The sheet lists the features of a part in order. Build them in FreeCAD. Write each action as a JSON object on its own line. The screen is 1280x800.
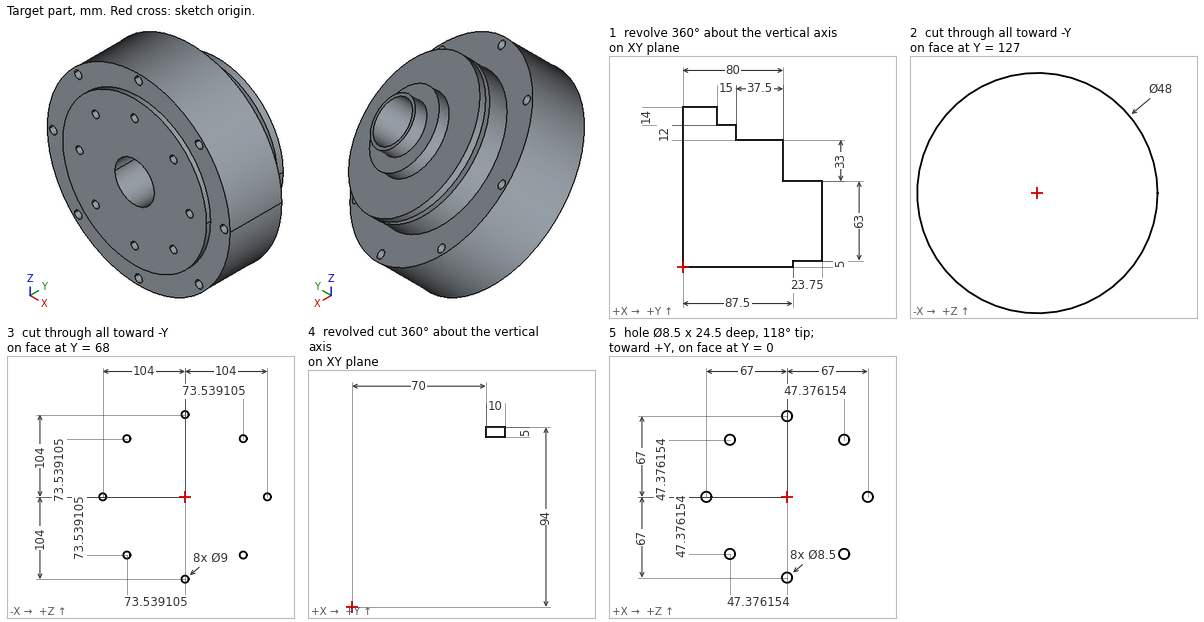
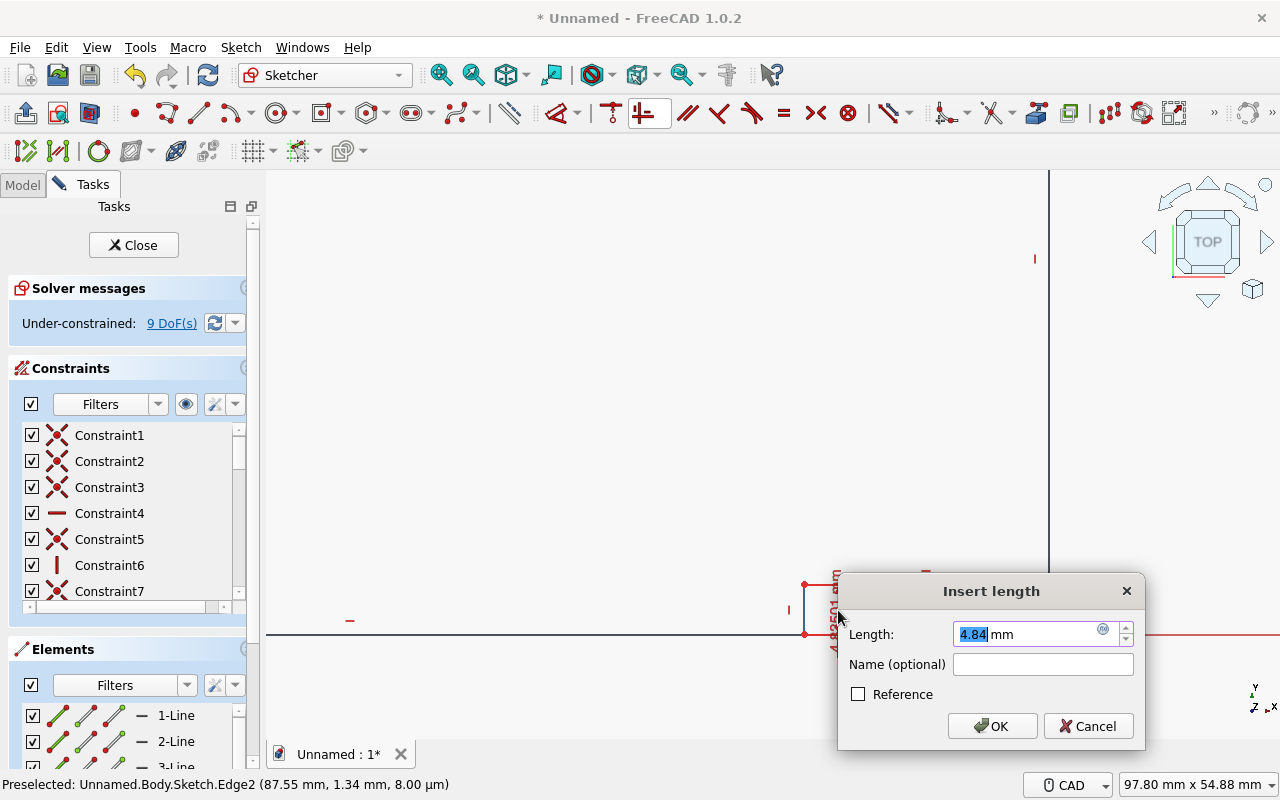
{"action": "type", "text": "5"}
{"action": "key", "text": "Return"}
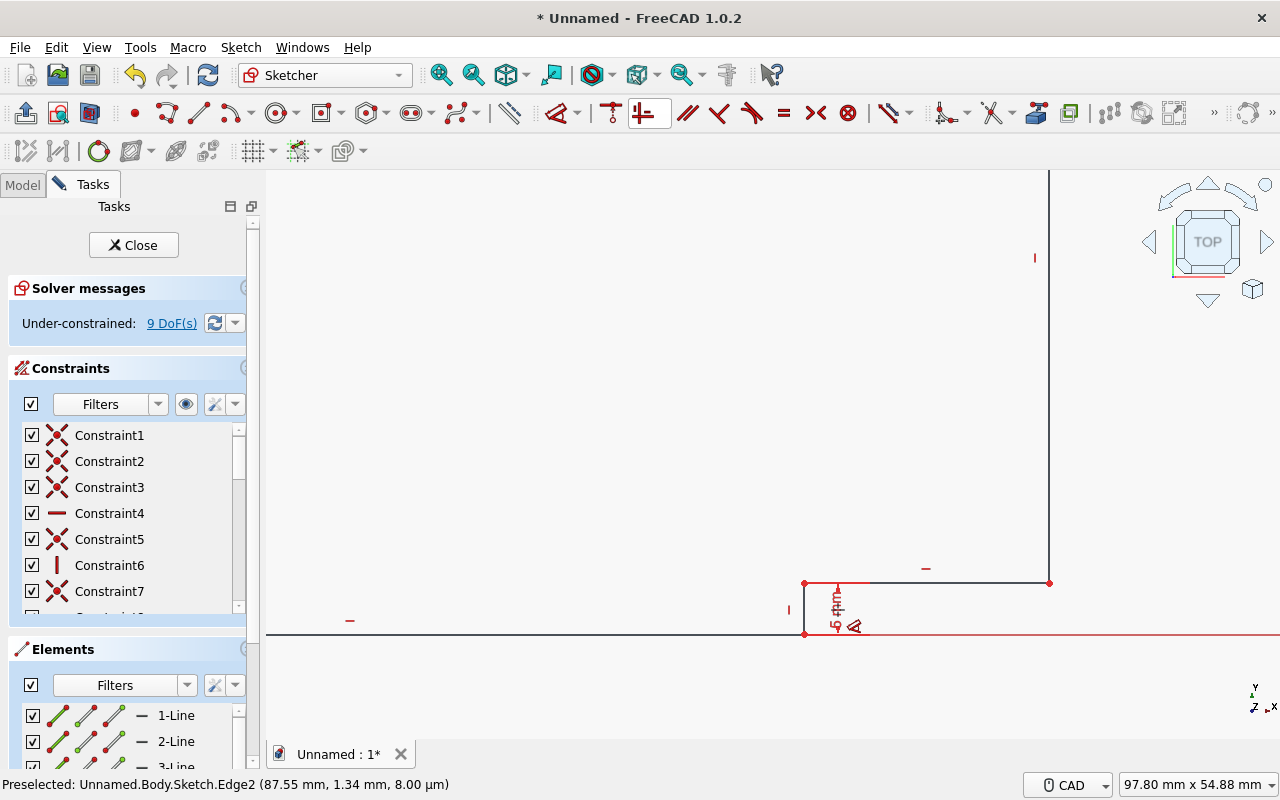
{"action": "scroll", "coordinate": [804, 660], "scroll_direction": "down", "scroll_amount": 6}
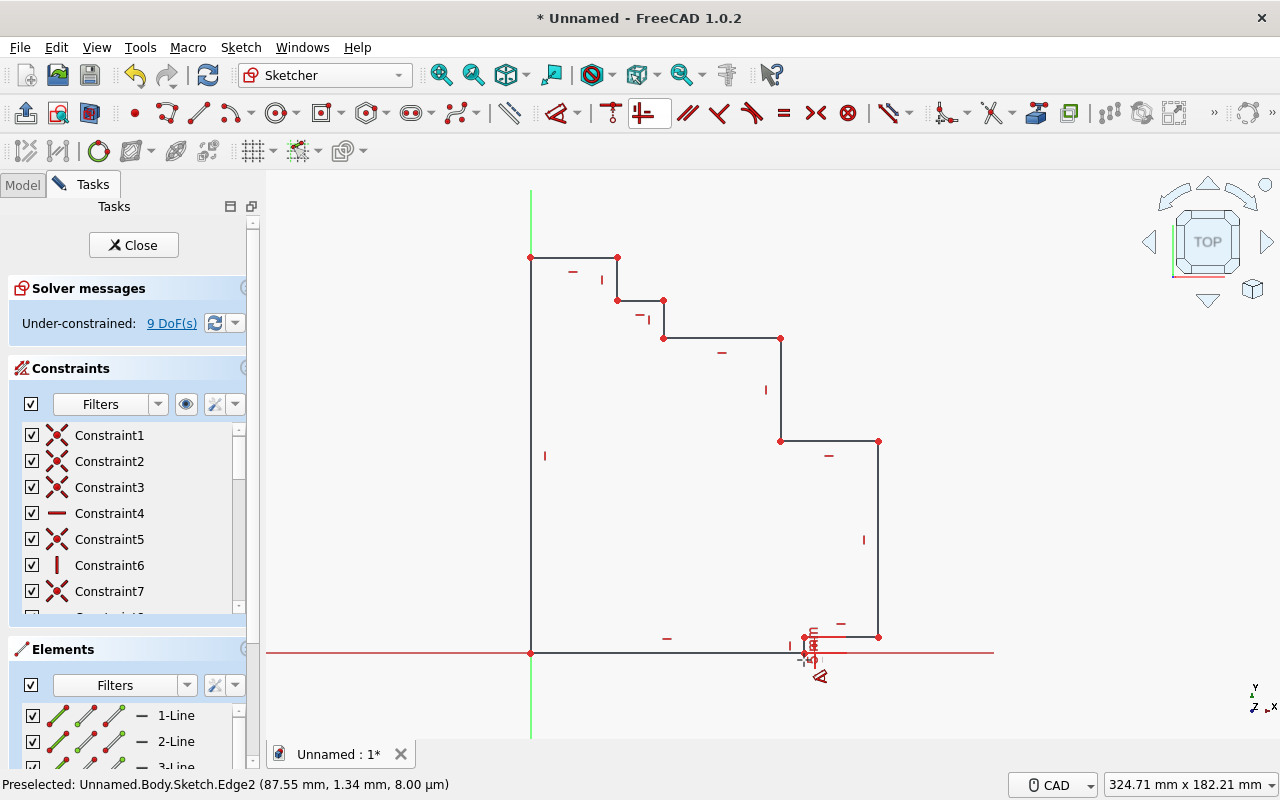
{"action": "left_click", "coordinate": [878, 579]}
{"action": "left_click", "coordinate": [912, 539]}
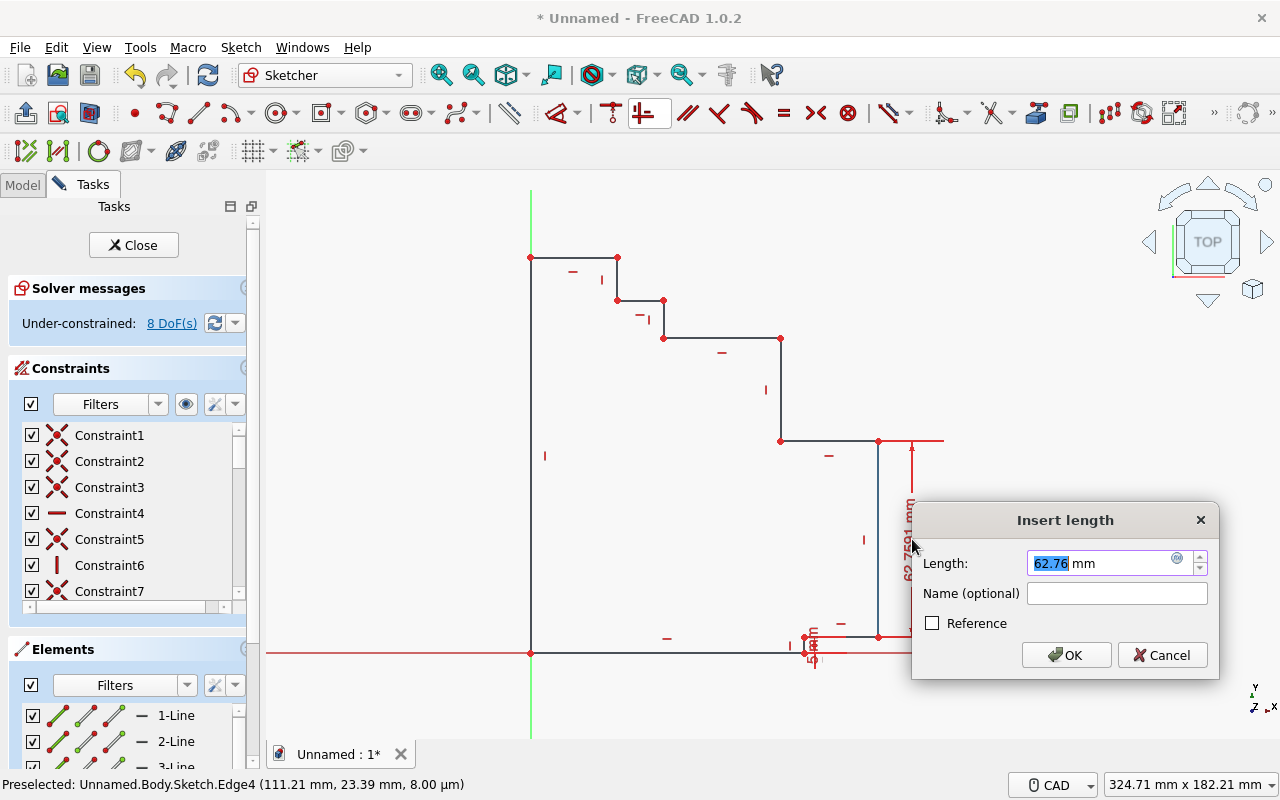
{"action": "type", "text": "63"}
{"action": "key", "text": "Return"}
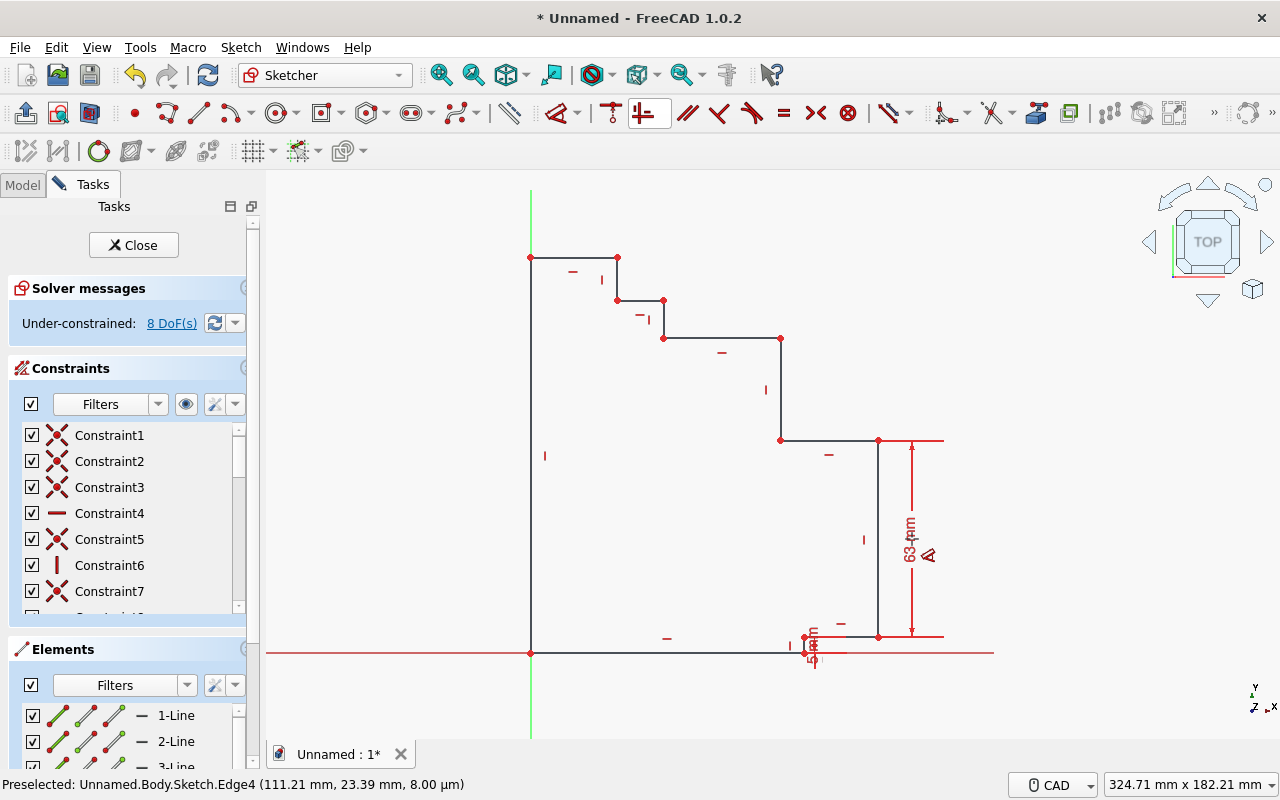
{"action": "left_click", "coordinate": [781, 410]}
{"action": "left_click", "coordinate": [815, 390]}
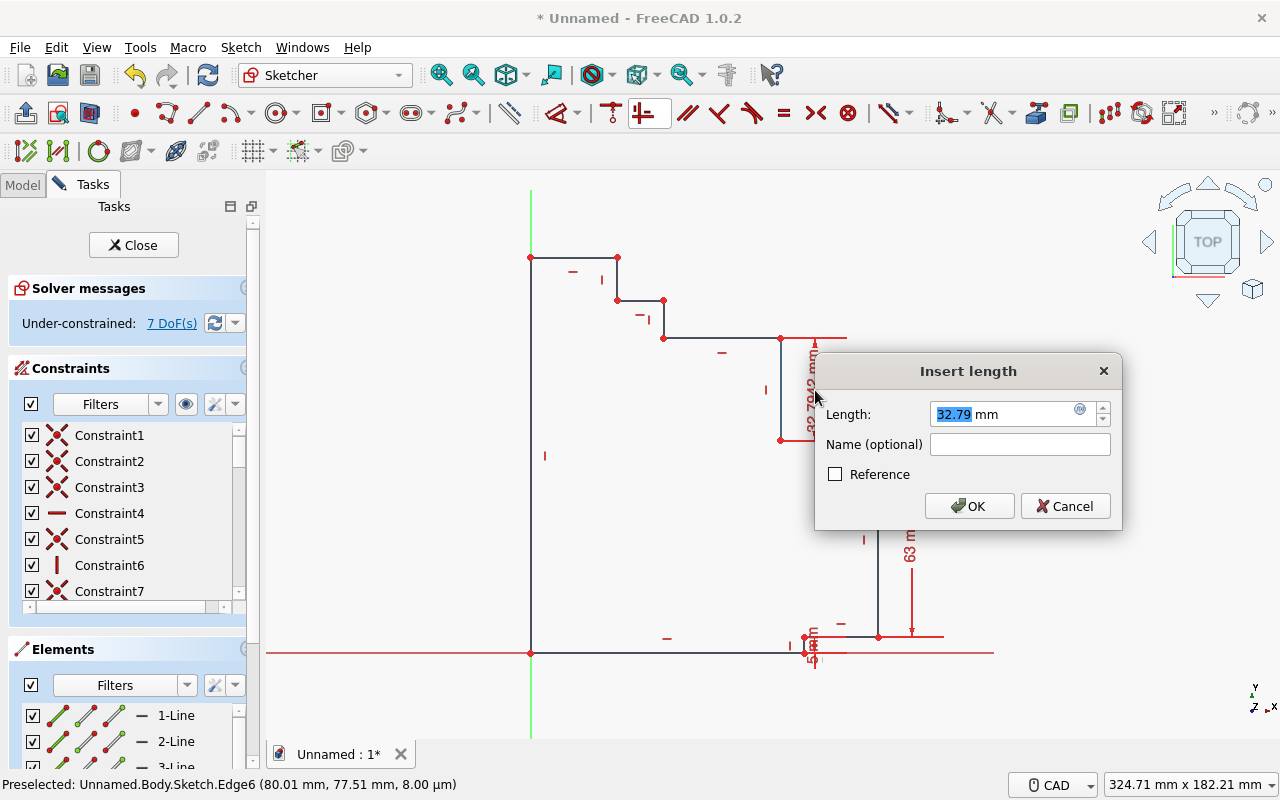
{"action": "type", "text": "33"}
{"action": "key", "text": "Return"}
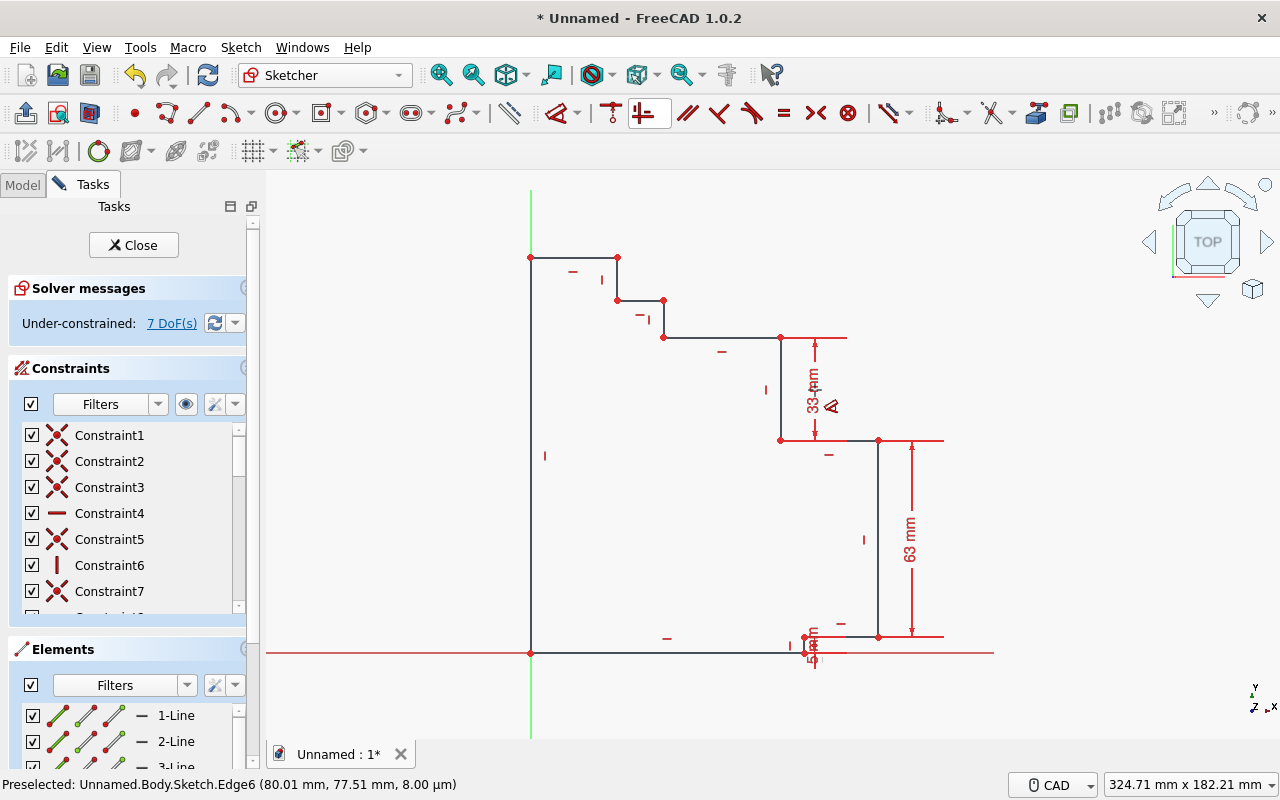
{"action": "scroll", "coordinate": [664, 327], "scroll_direction": "up", "scroll_amount": 2}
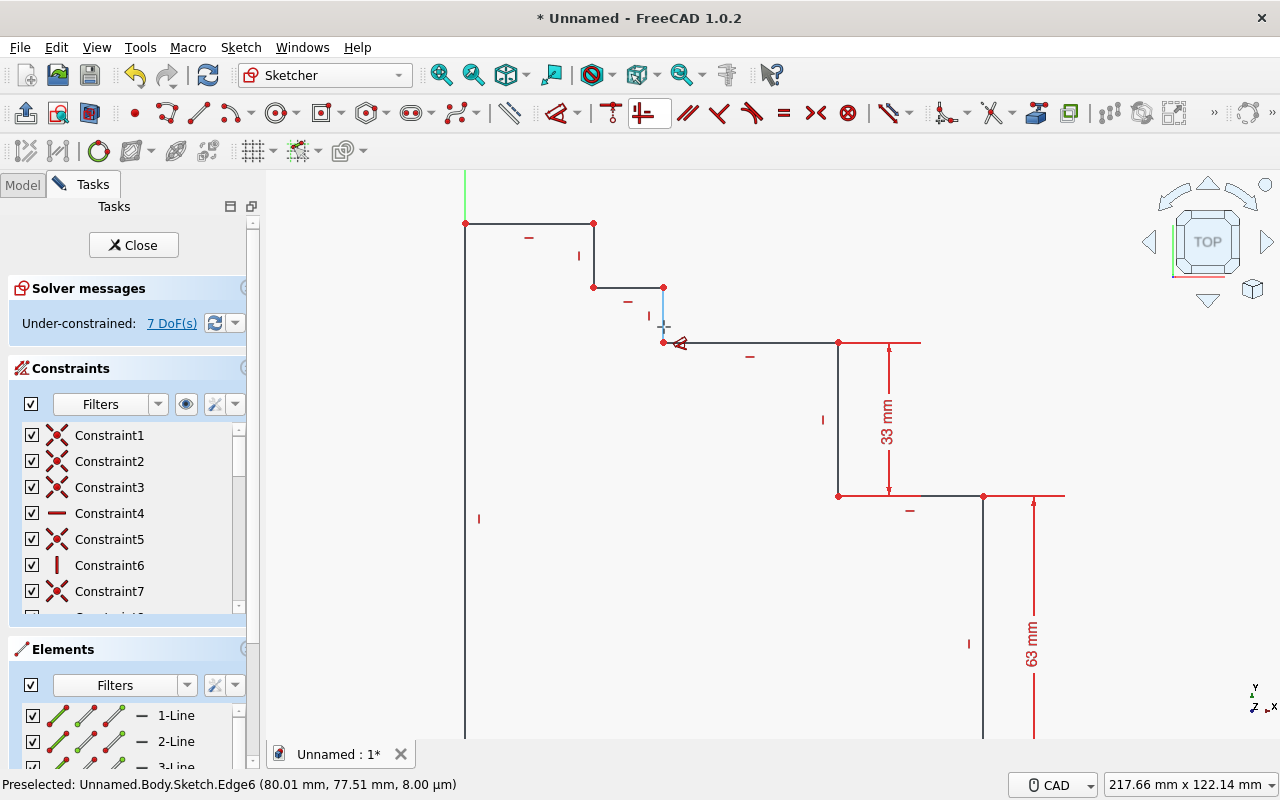
{"action": "left_click", "coordinate": [663, 326]}
{"action": "left_click", "coordinate": [629, 315]}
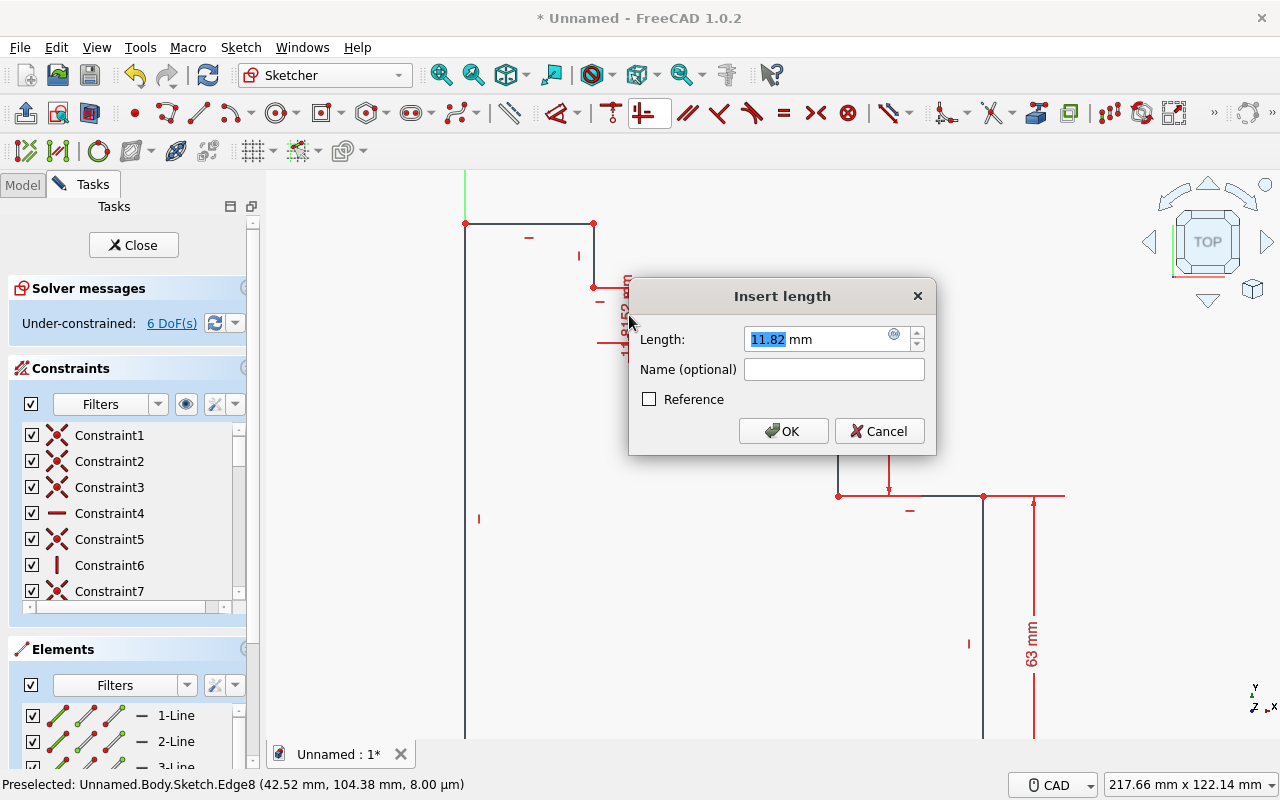
{"action": "type", "text": "12"}
{"action": "key", "text": "Return"}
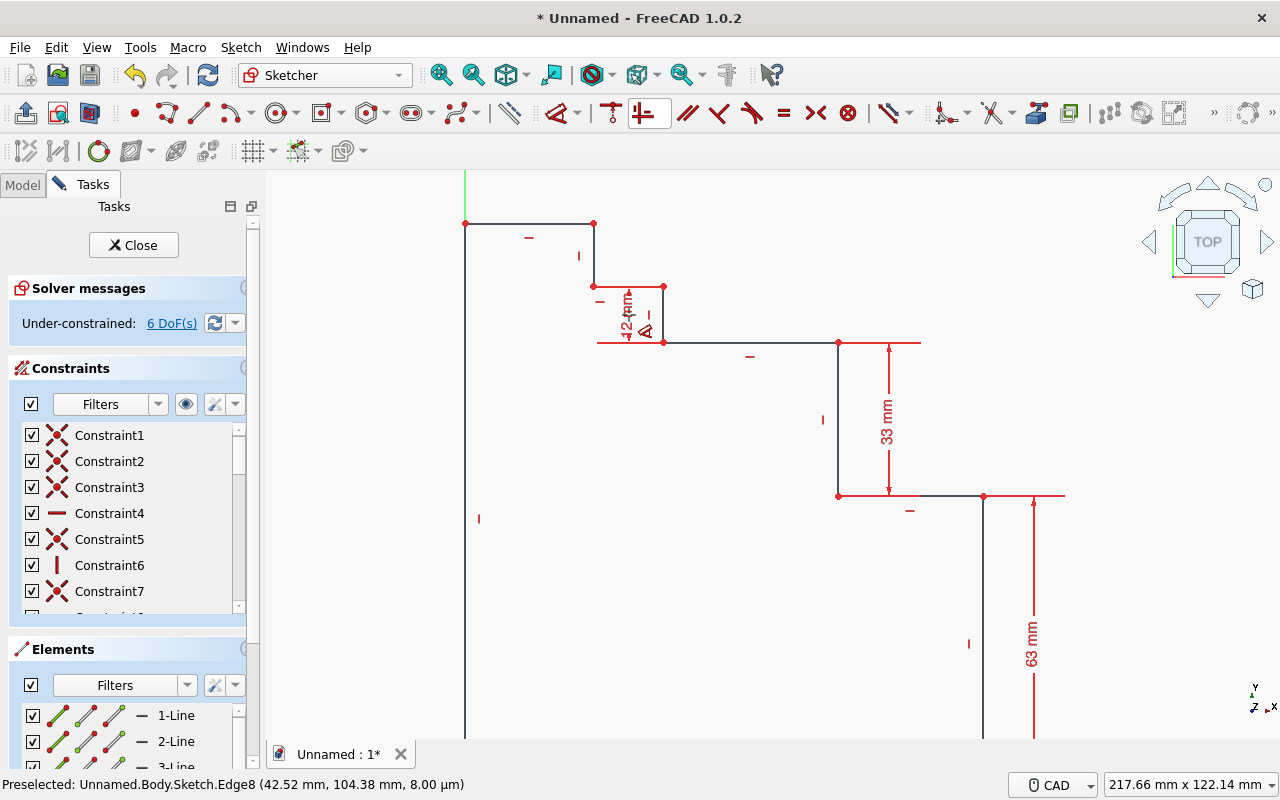
{"action": "left_click", "coordinate": [643, 287]}
{"action": "left_click", "coordinate": [629, 253]}